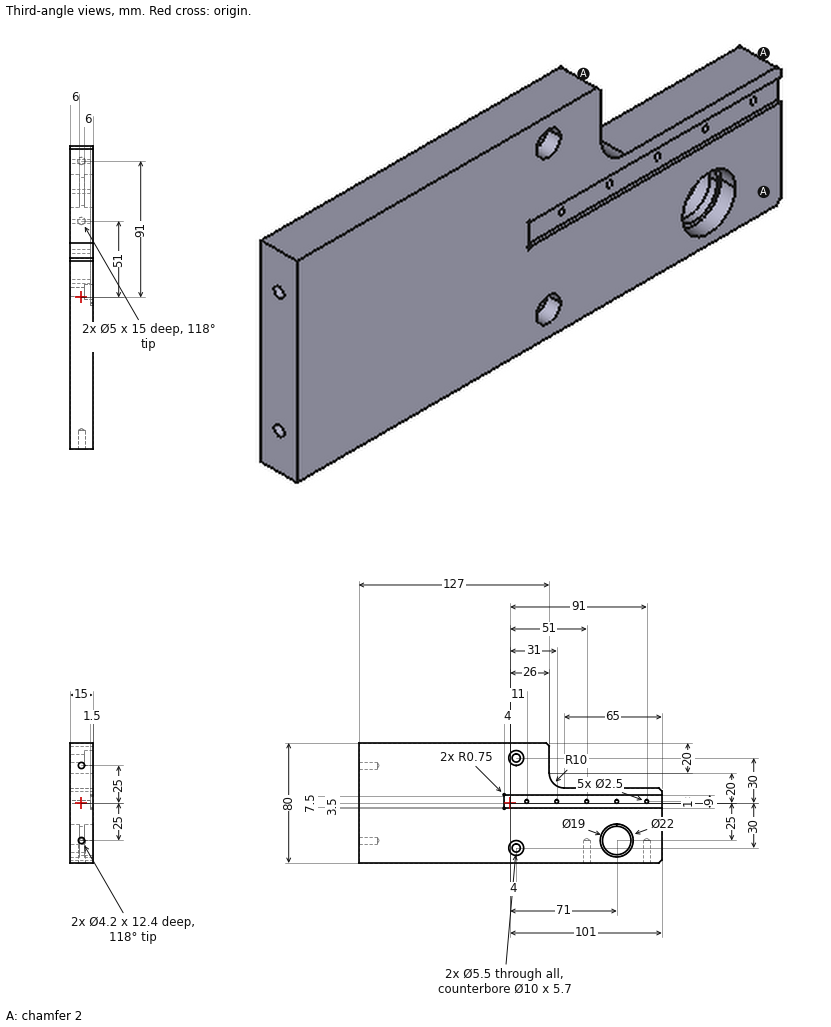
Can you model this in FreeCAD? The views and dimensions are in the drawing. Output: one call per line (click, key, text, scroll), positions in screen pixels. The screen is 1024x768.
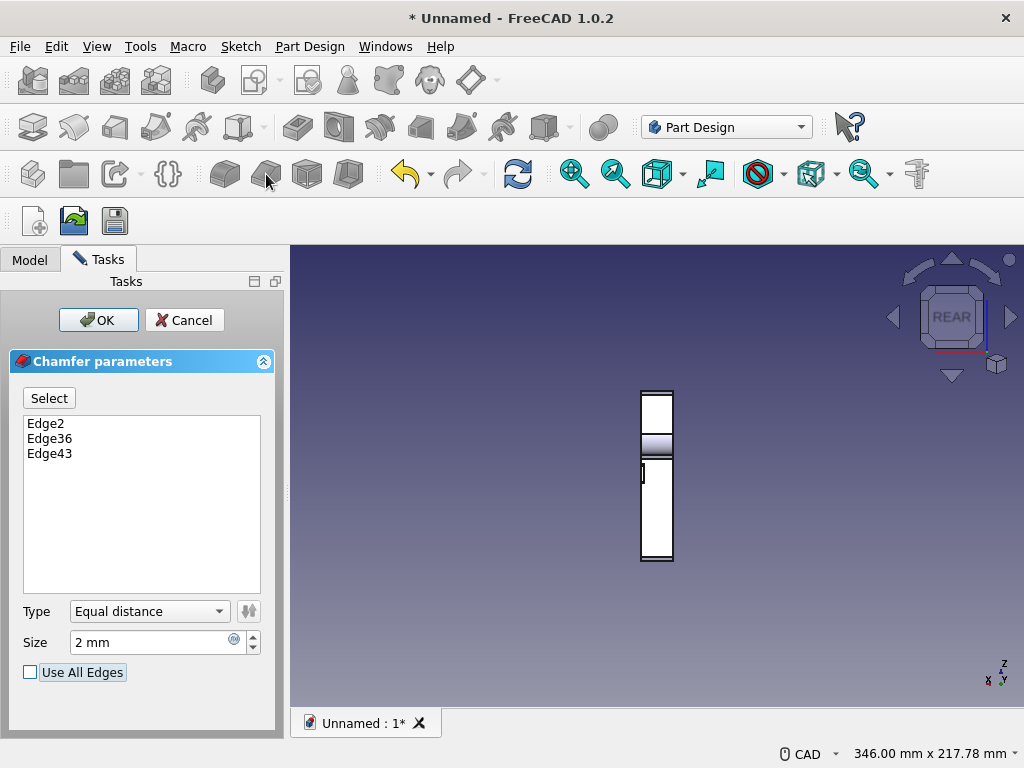
click(99, 320)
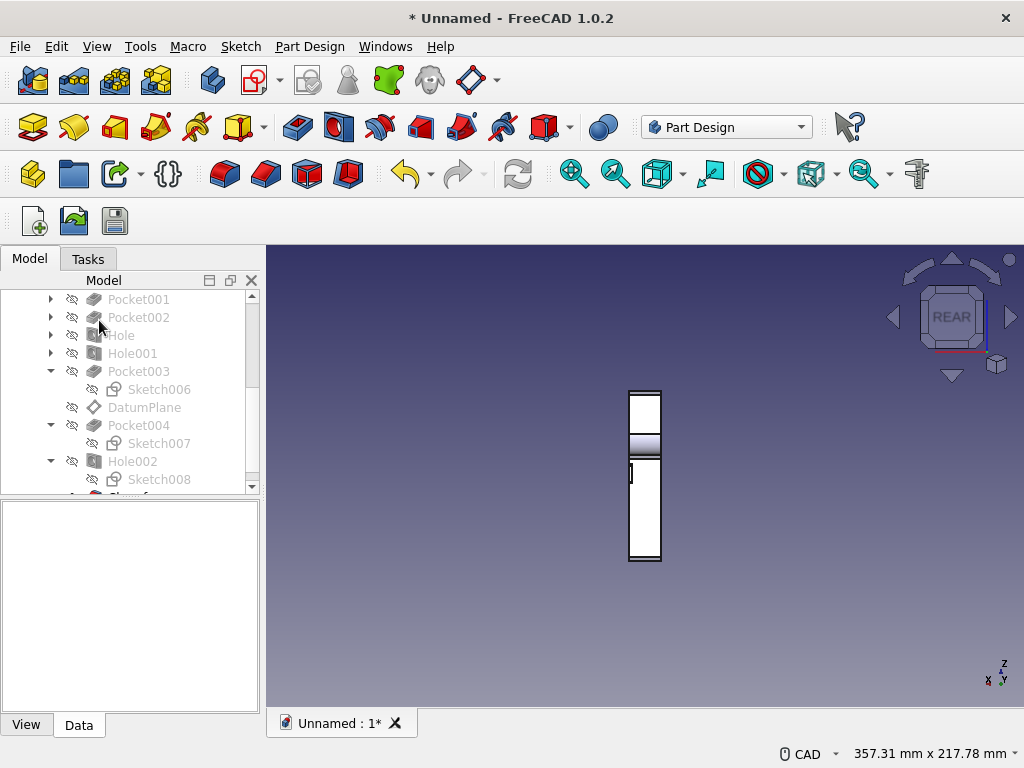
key(0)